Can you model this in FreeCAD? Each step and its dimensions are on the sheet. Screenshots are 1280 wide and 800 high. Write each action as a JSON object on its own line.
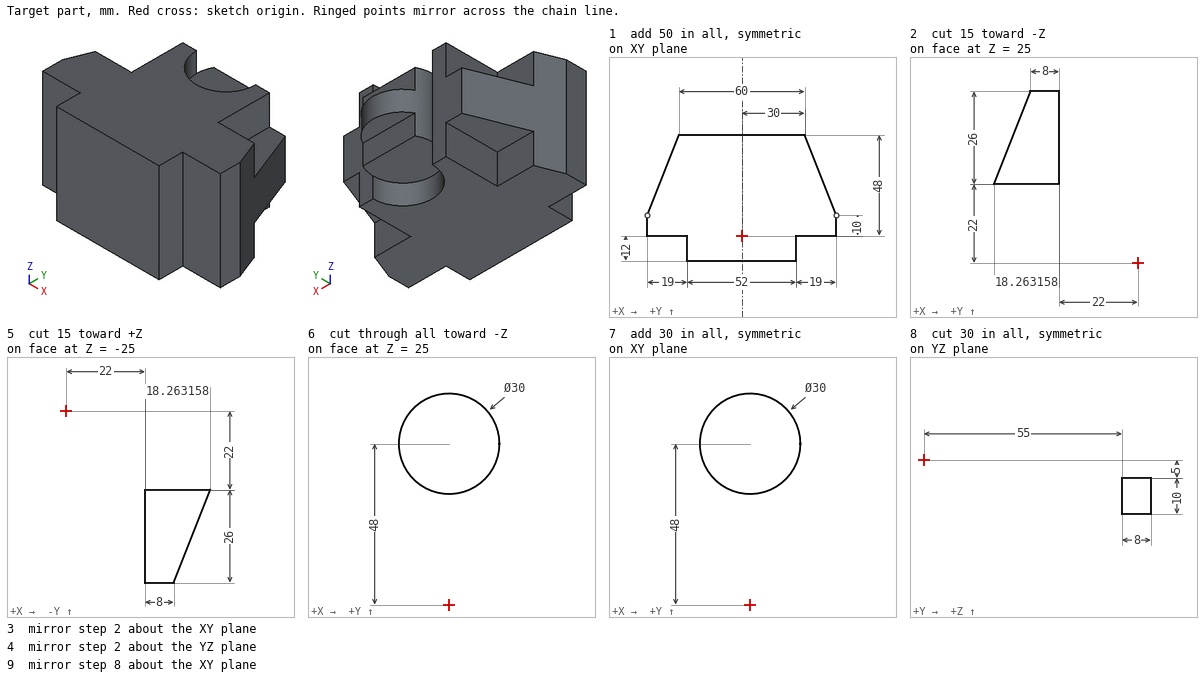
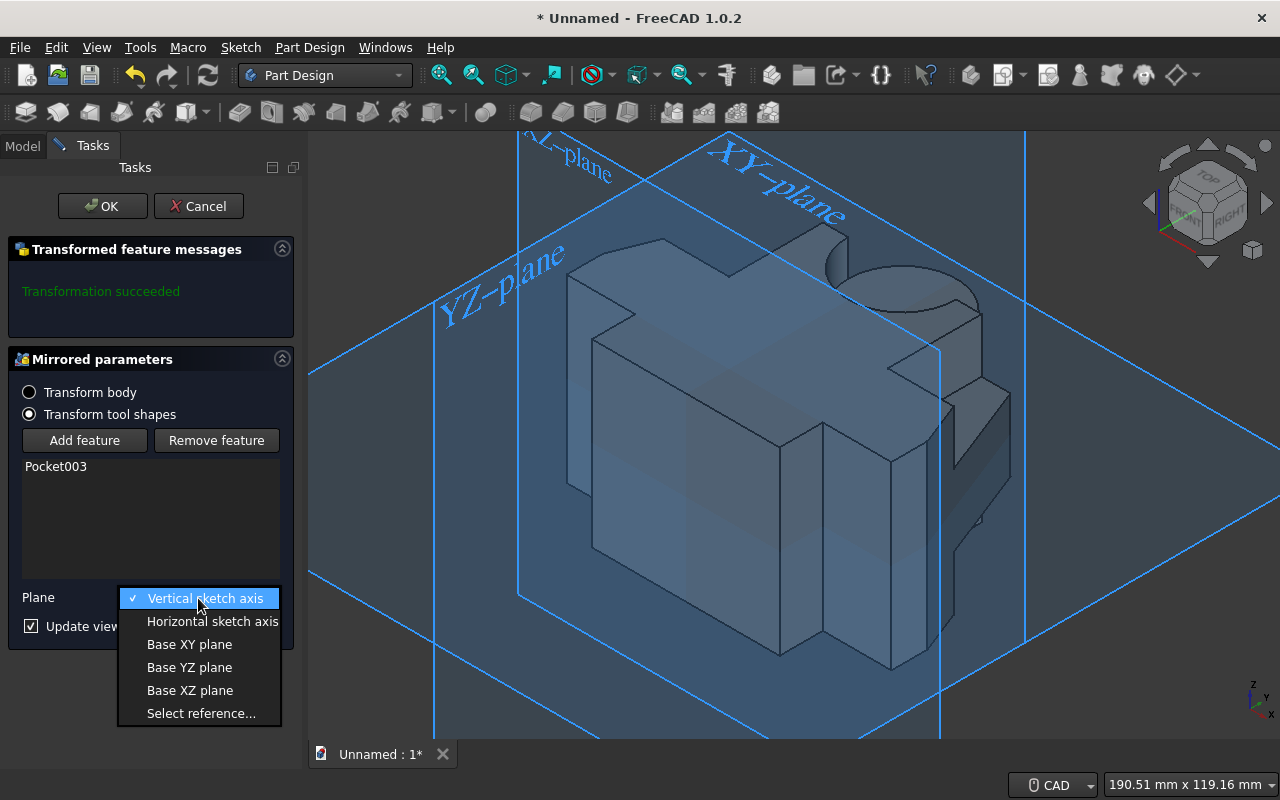
{"action": "left_click", "coordinate": [198, 644]}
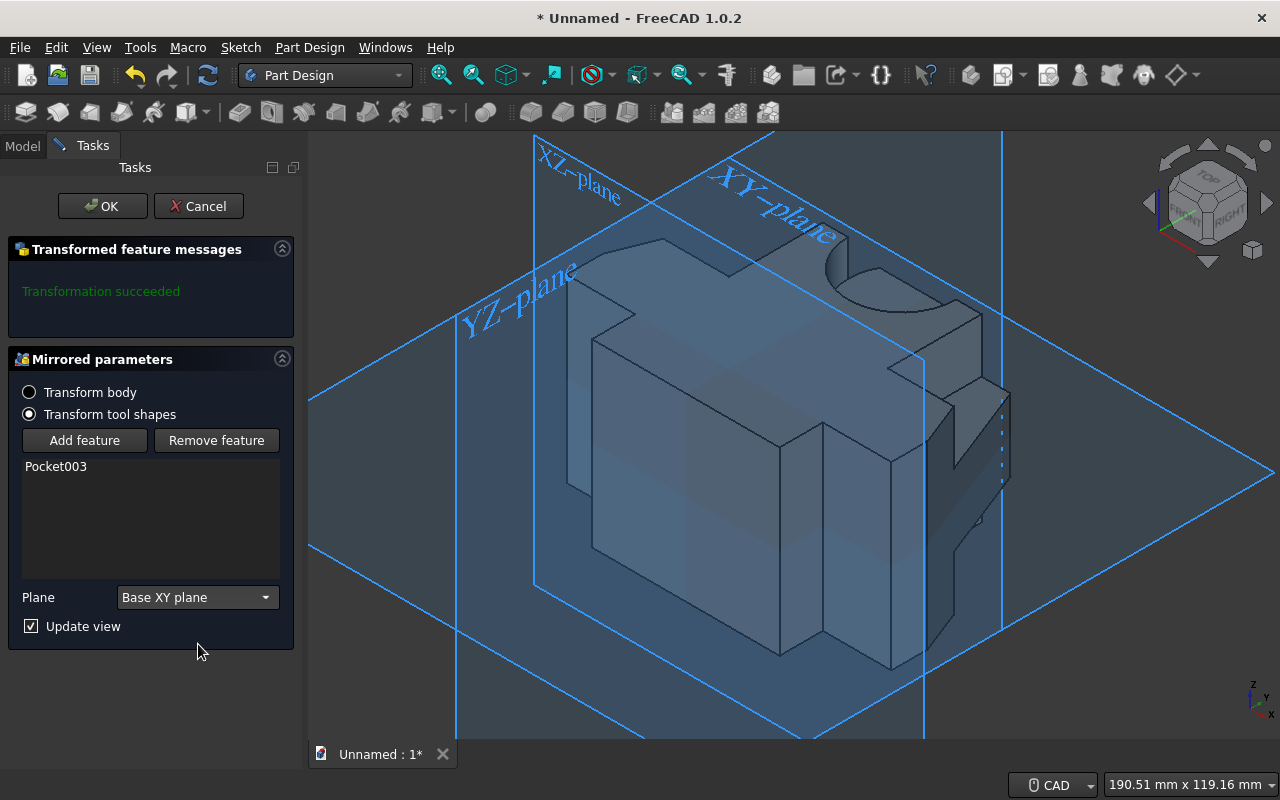
{"action": "left_click", "coordinate": [103, 206]}